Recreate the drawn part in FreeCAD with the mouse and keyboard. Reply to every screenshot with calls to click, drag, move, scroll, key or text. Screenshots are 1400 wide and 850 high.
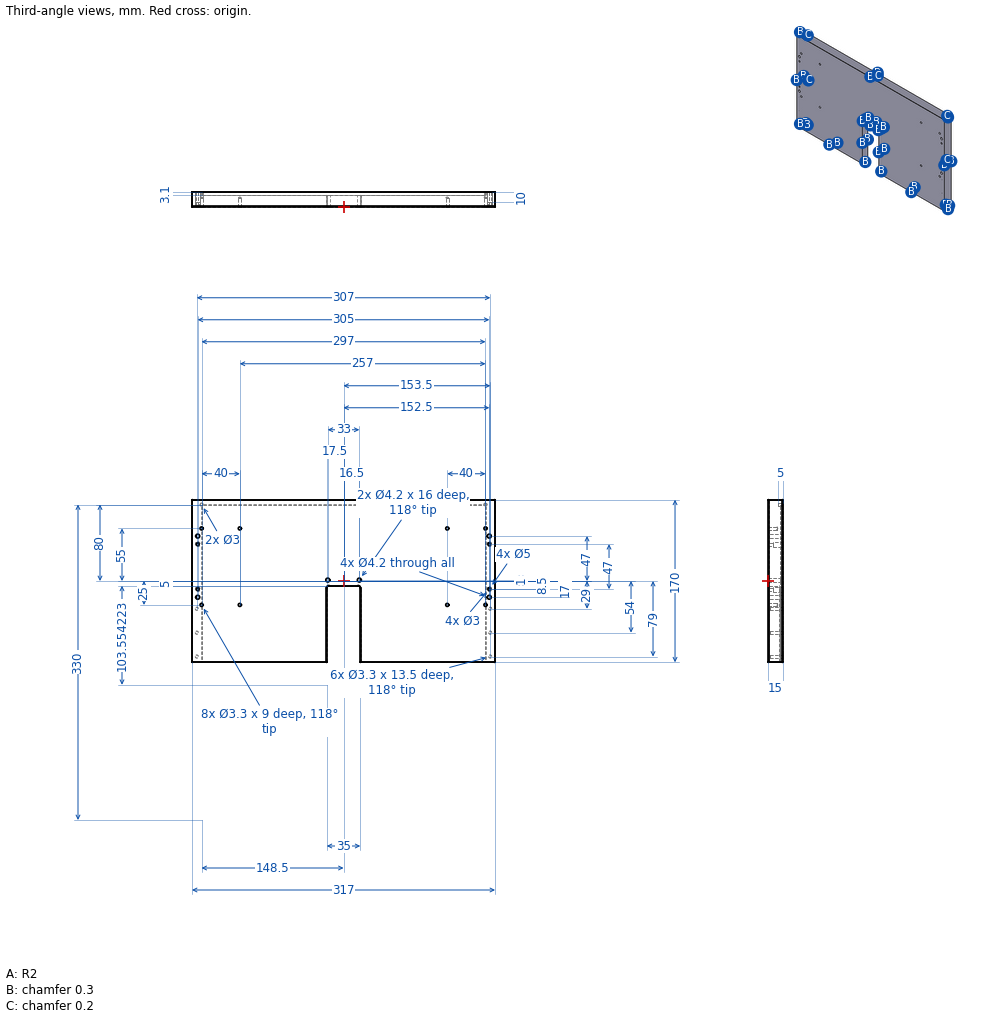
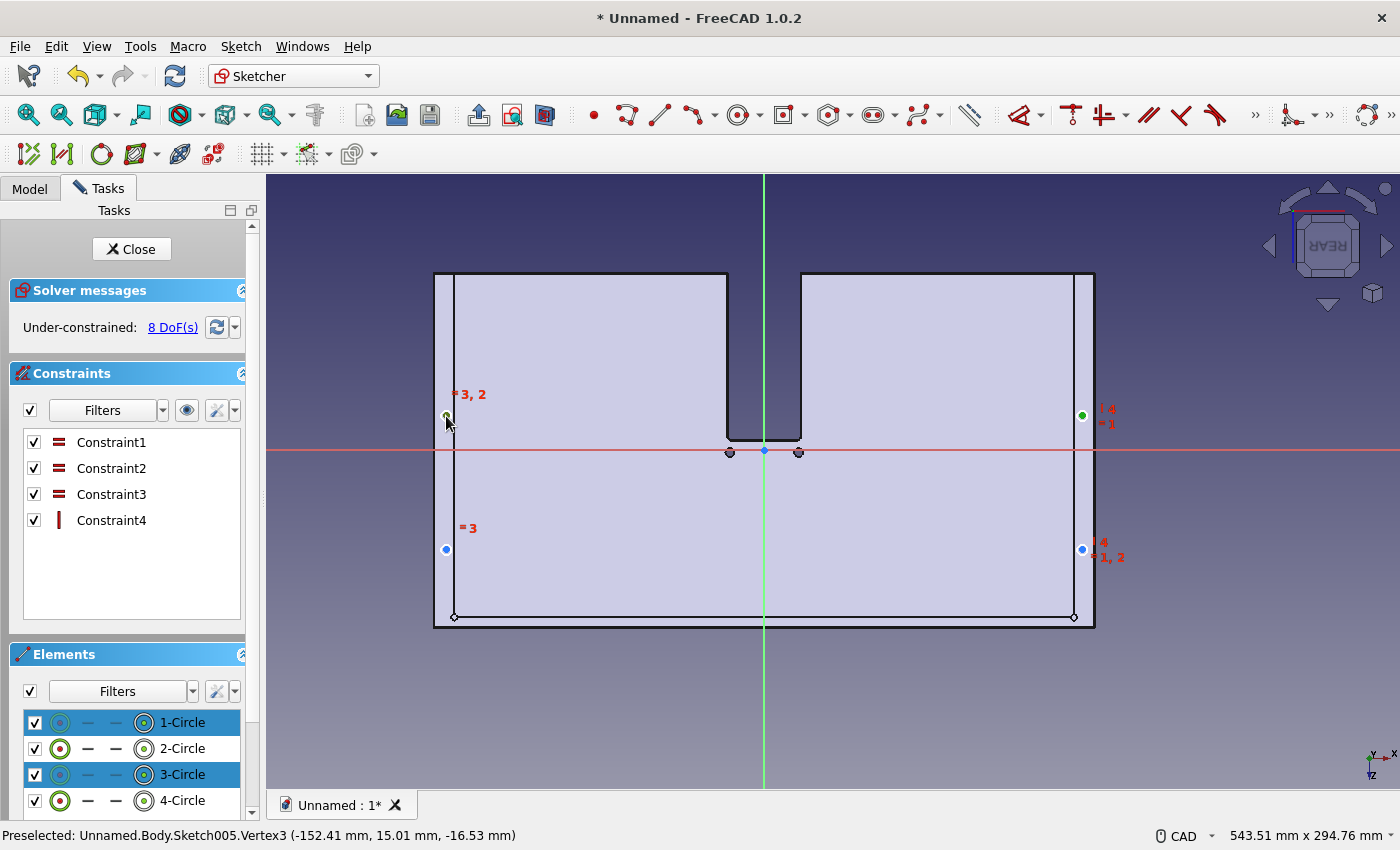
key(h)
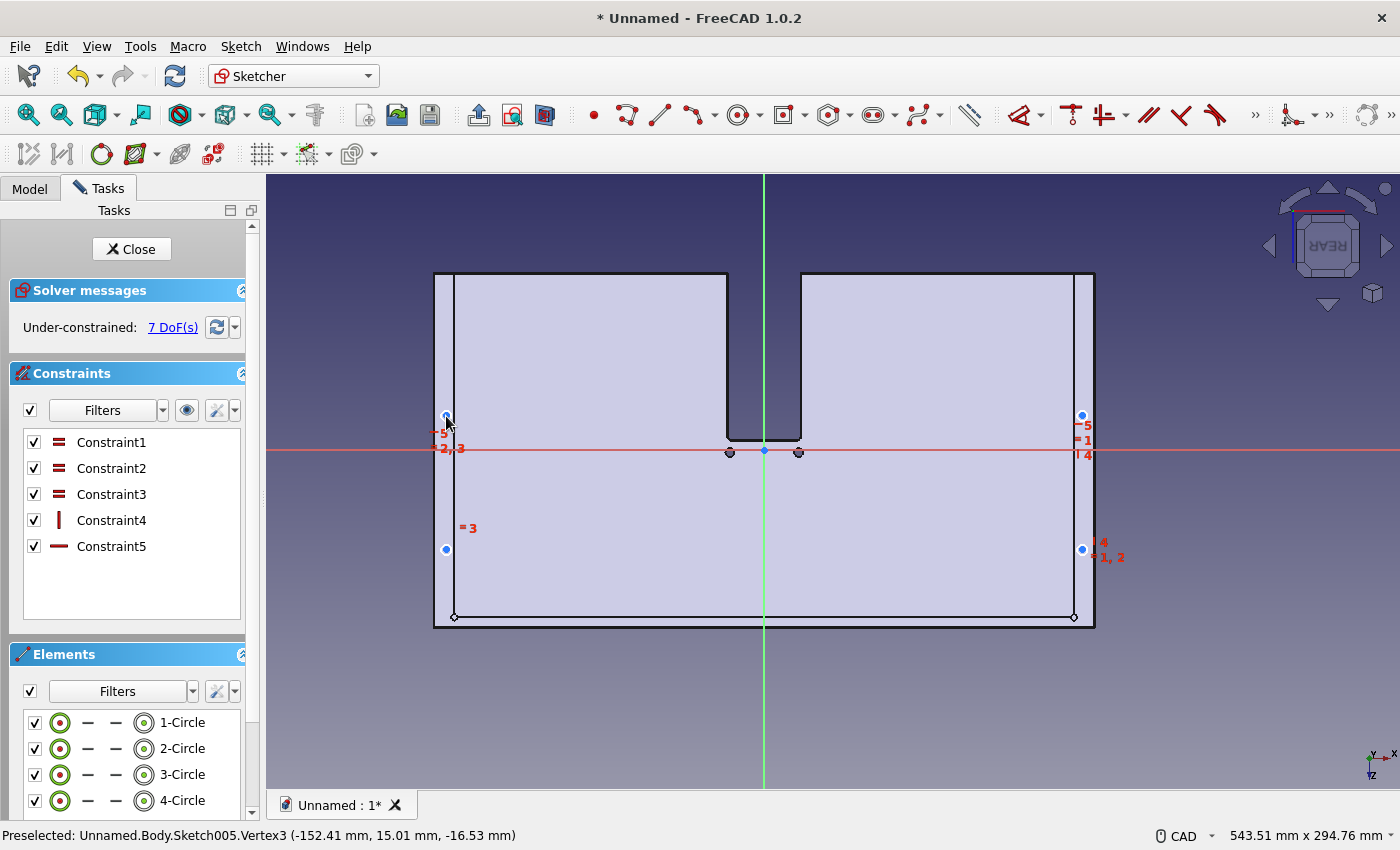
click(446, 416)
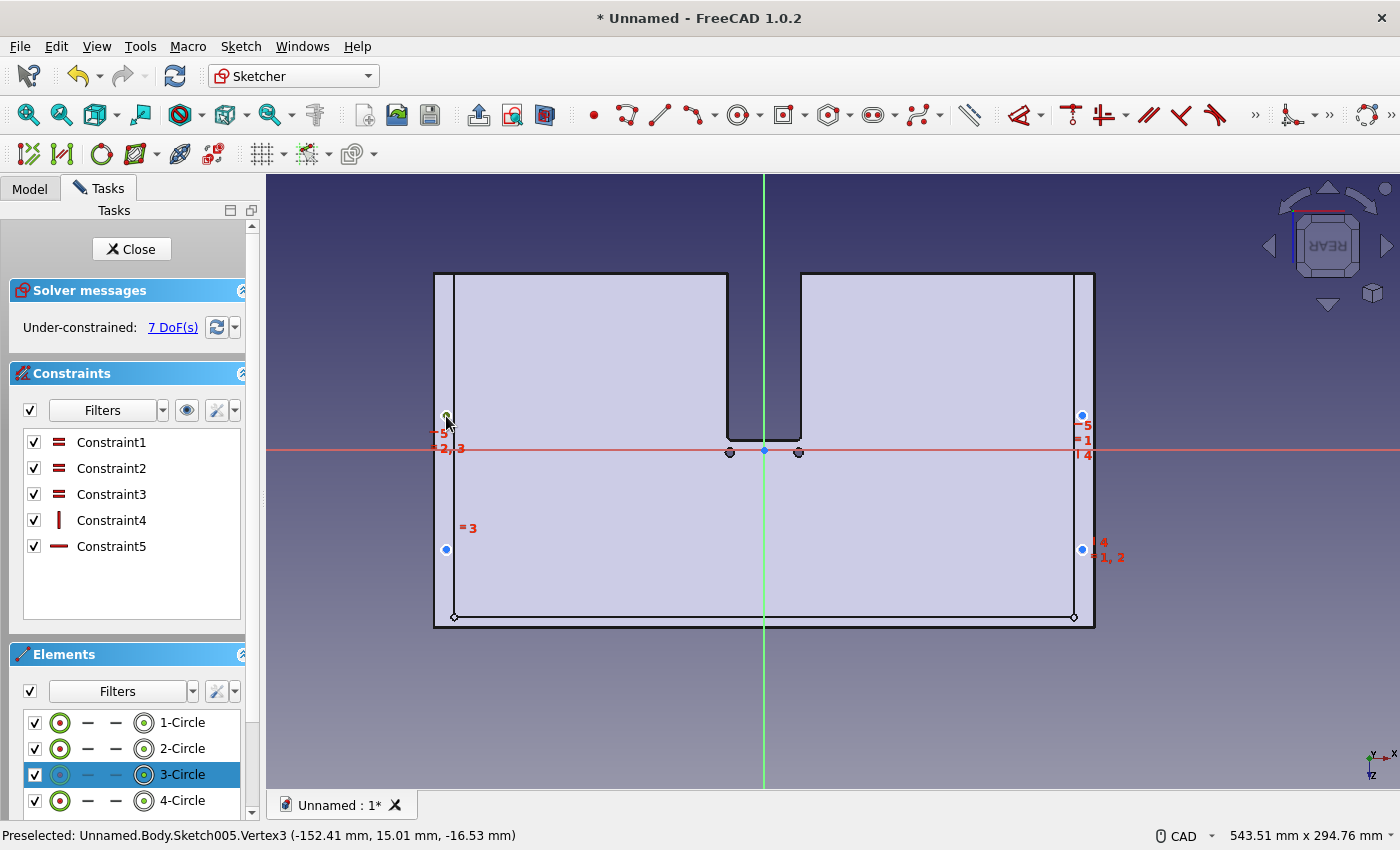
click(446, 550)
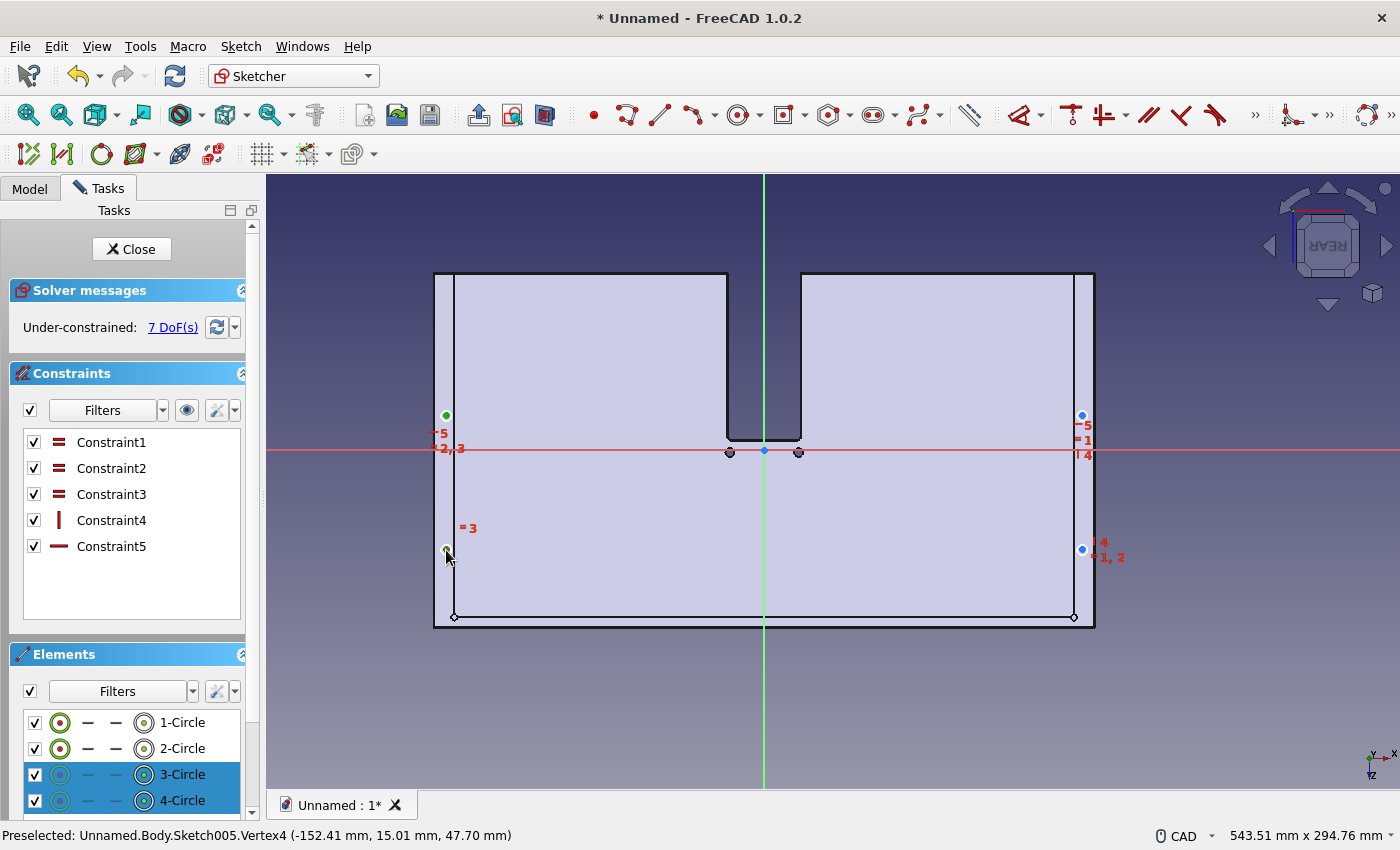
key(v)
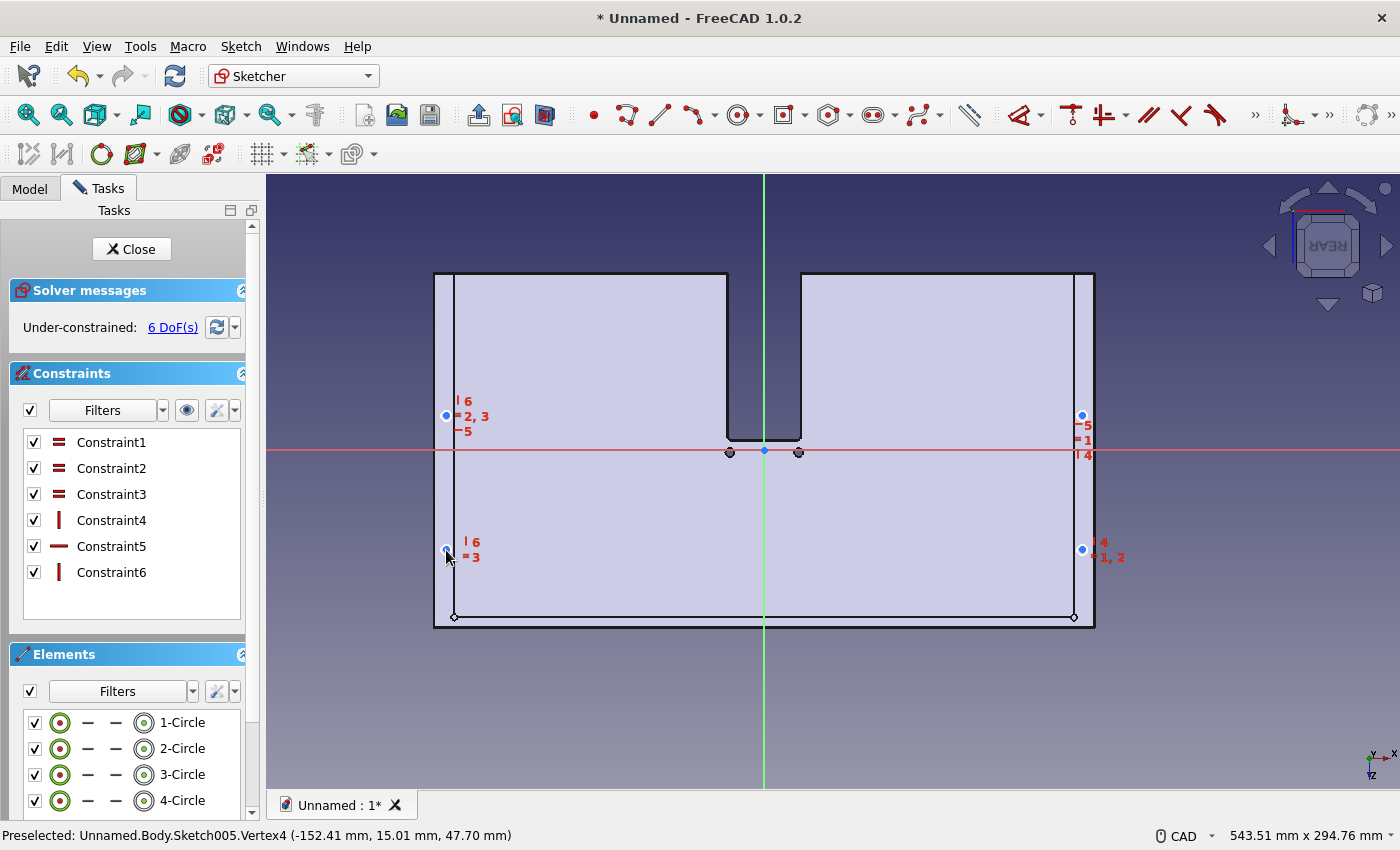
click(1082, 550)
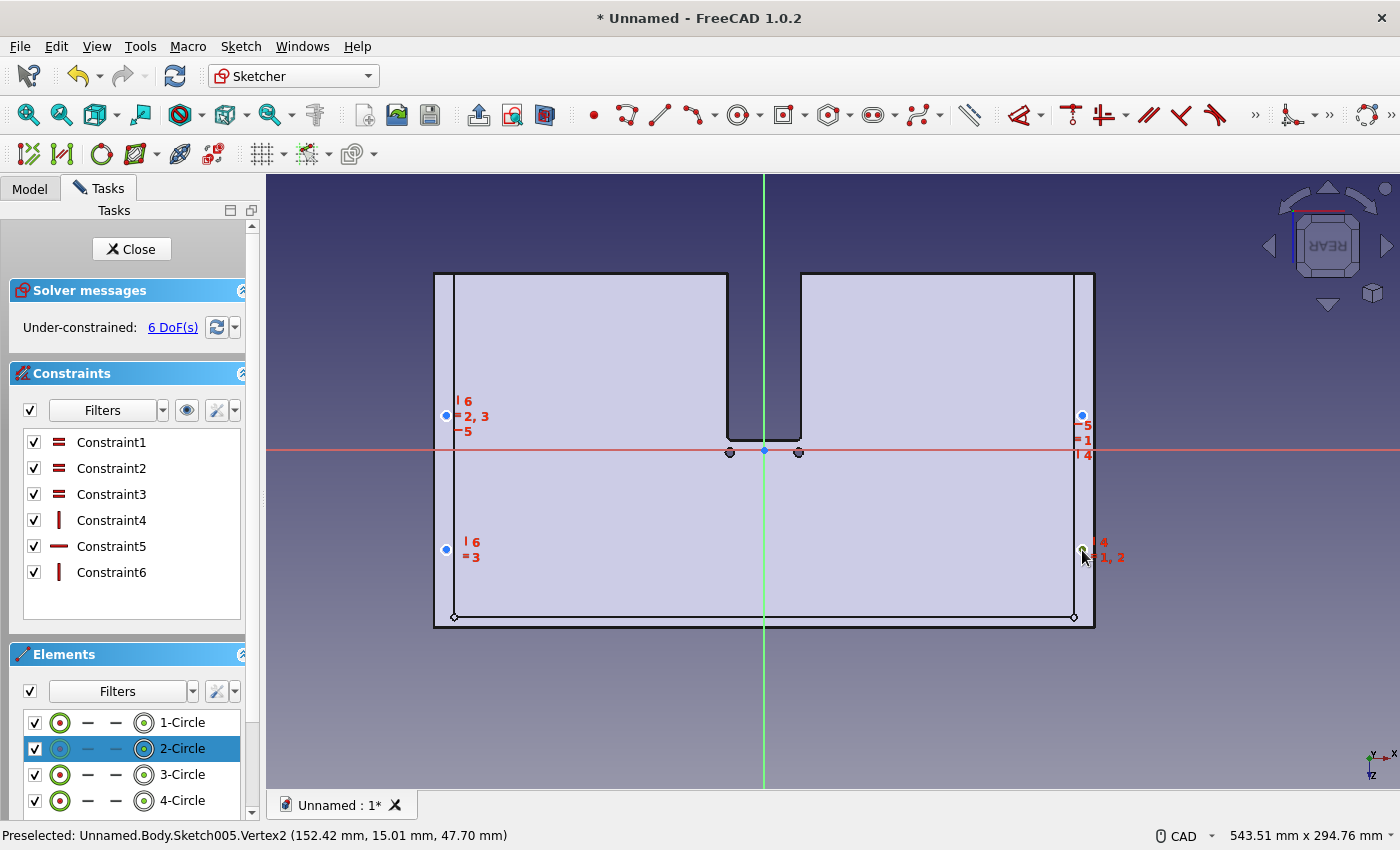
click(446, 550)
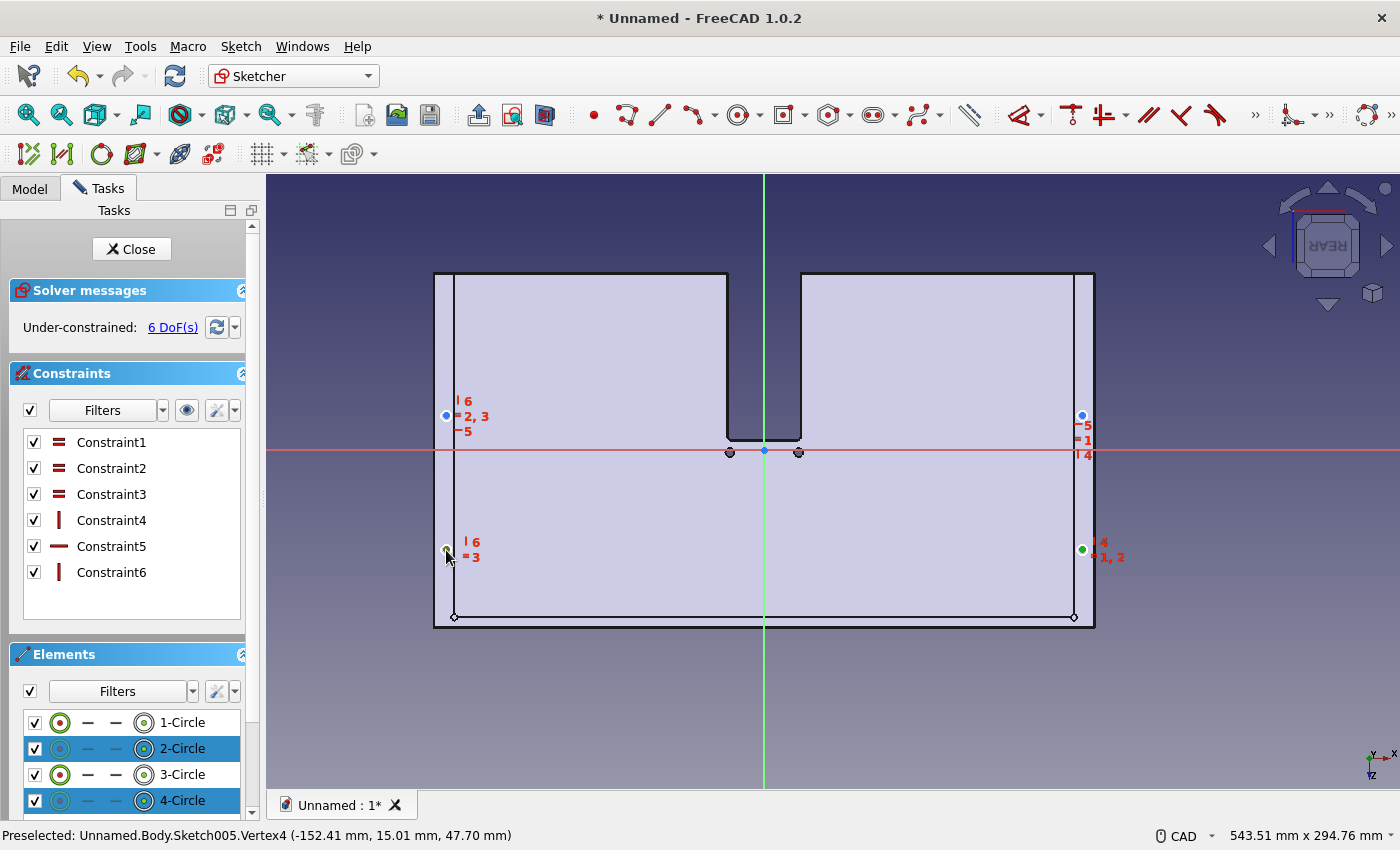
click(1126, 116)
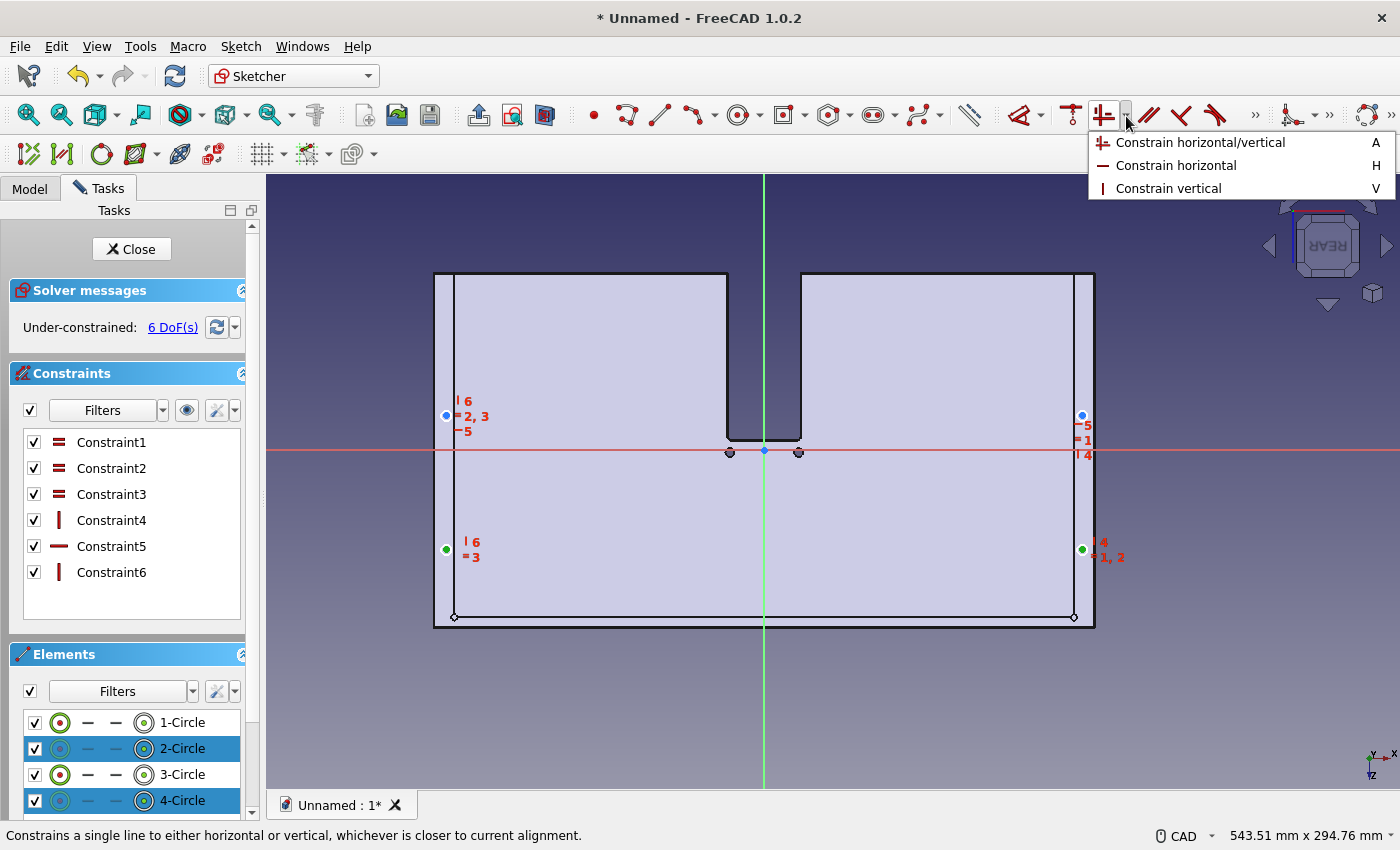
click(1242, 166)